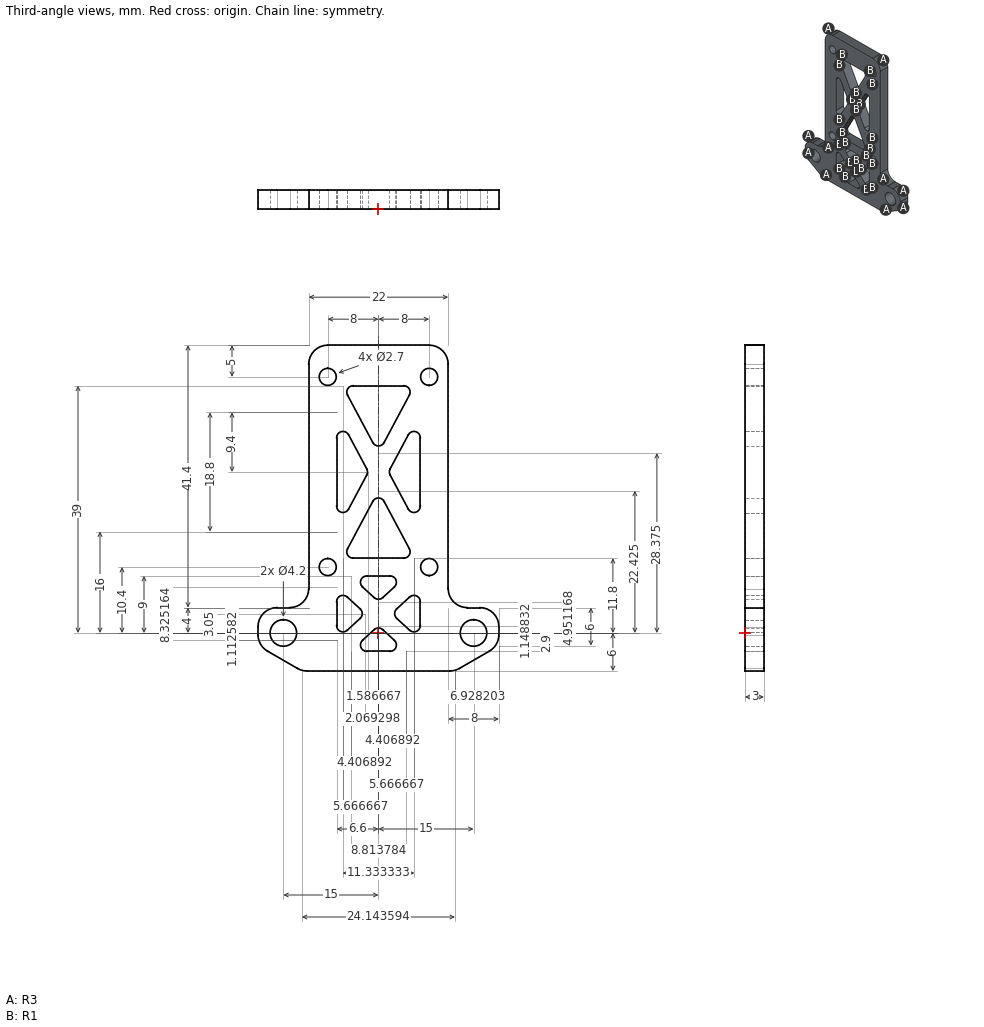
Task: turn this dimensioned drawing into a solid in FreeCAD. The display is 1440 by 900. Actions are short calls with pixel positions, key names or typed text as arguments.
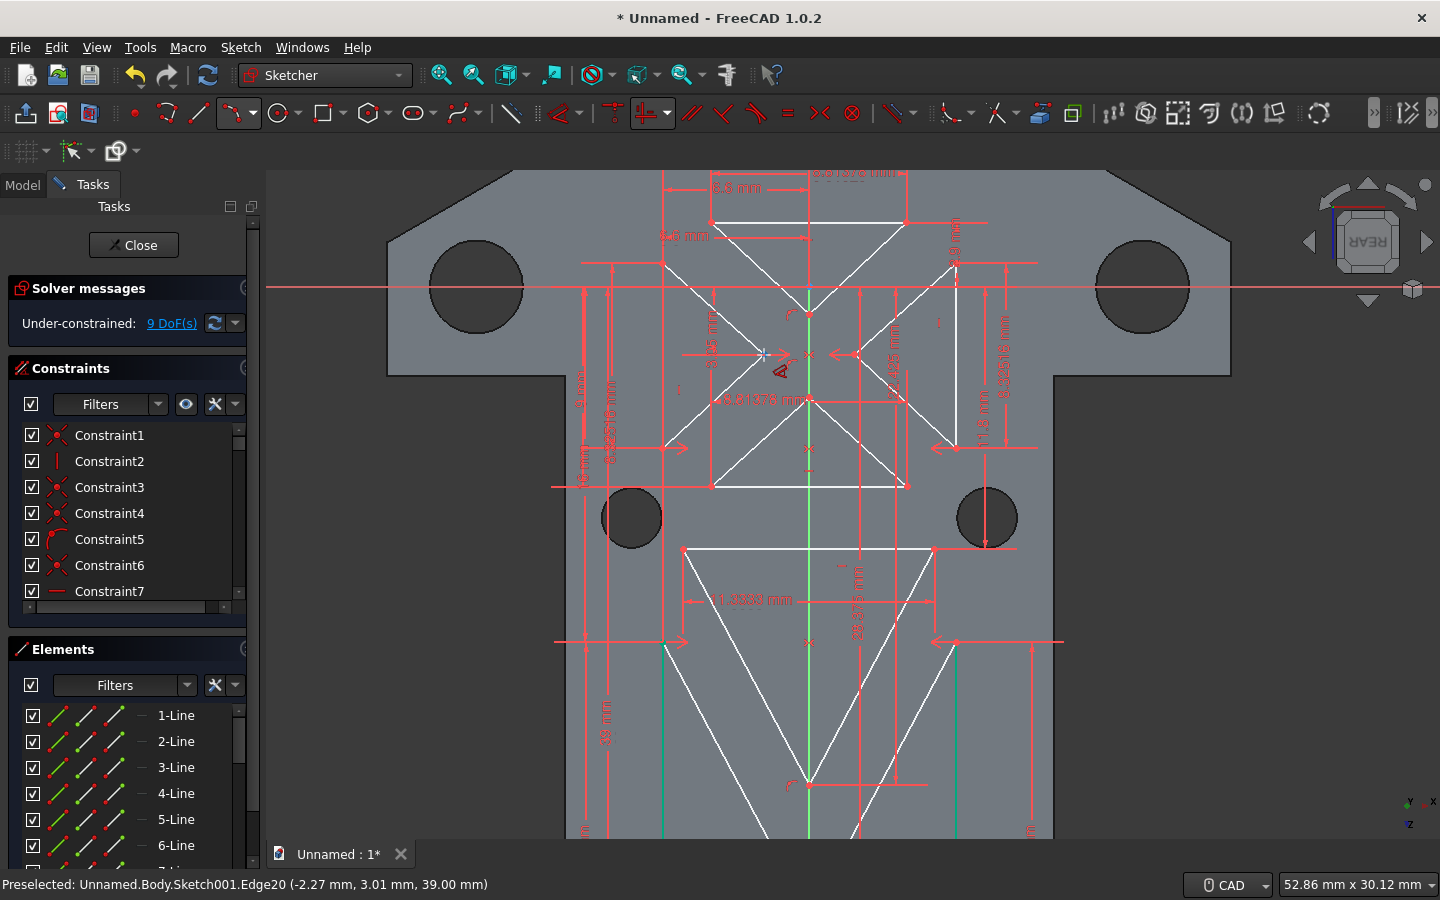
click(764, 355)
click(787, 253)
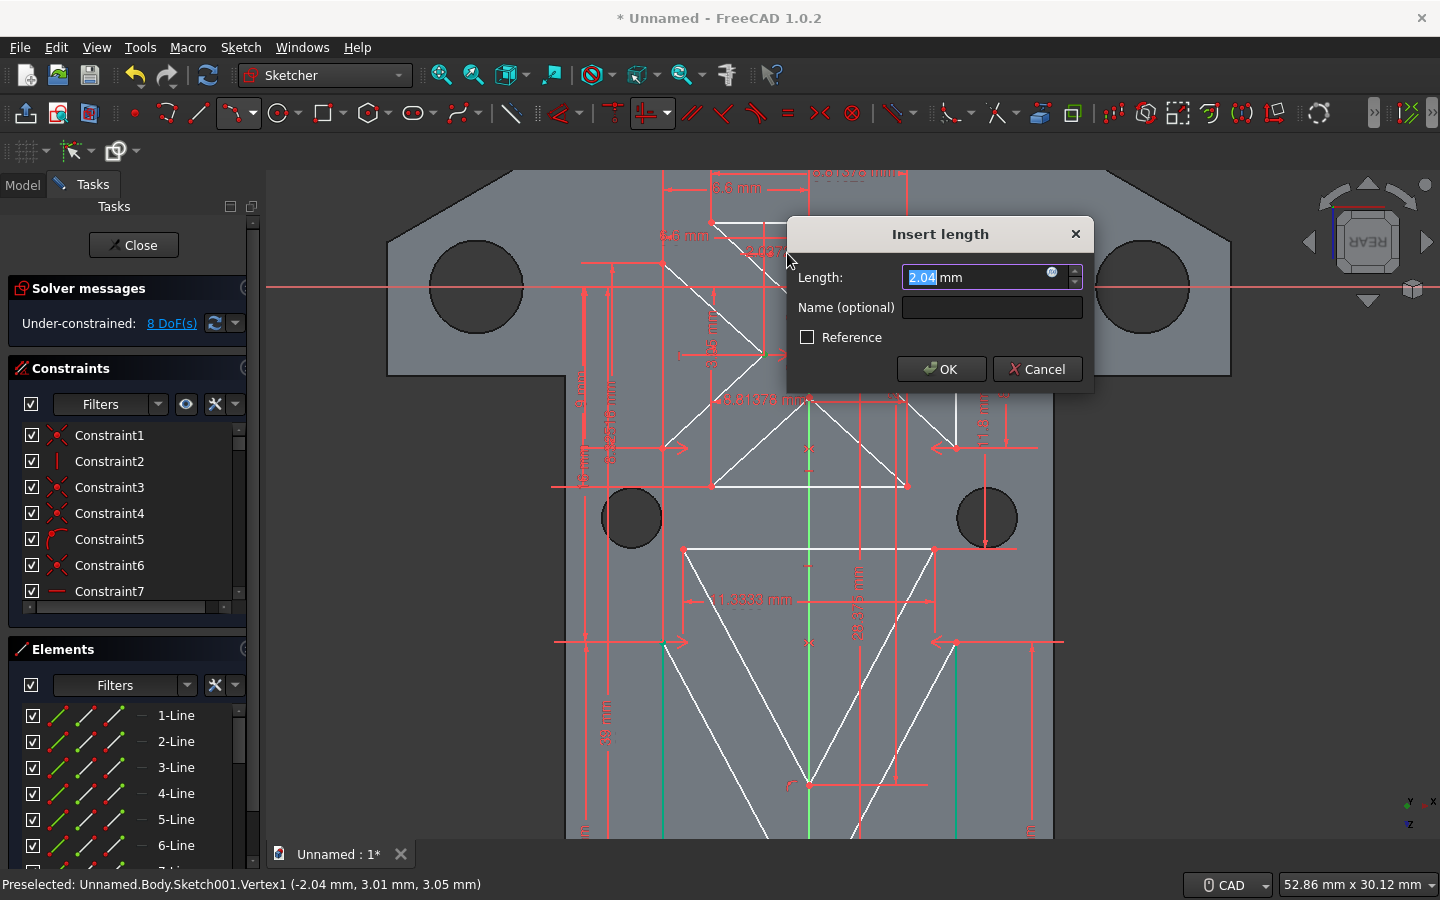
text(2.069298)
key(Return)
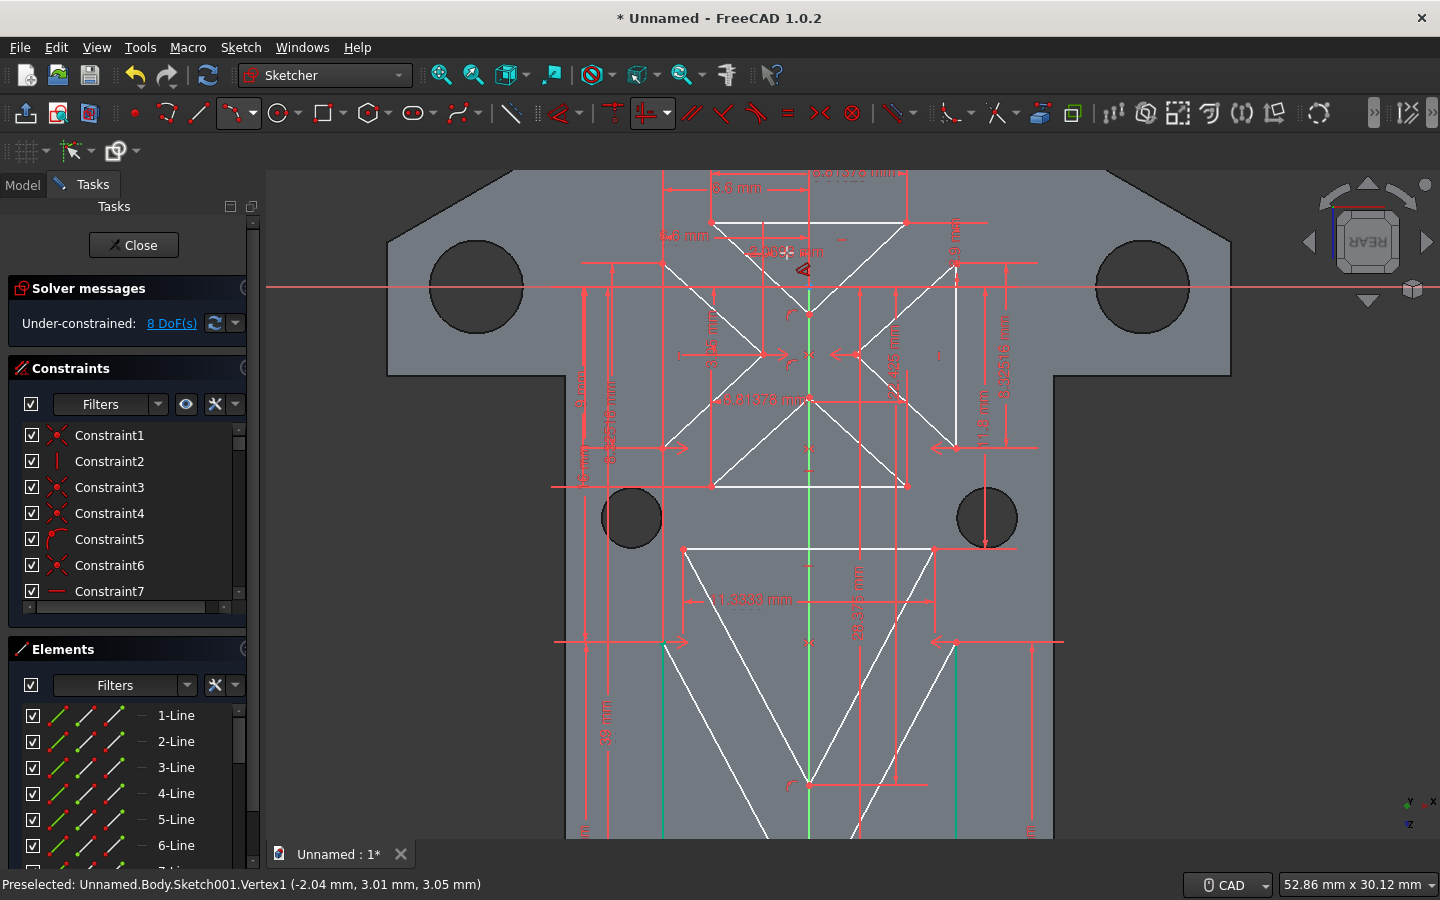
scroll(663, 263, up, 3)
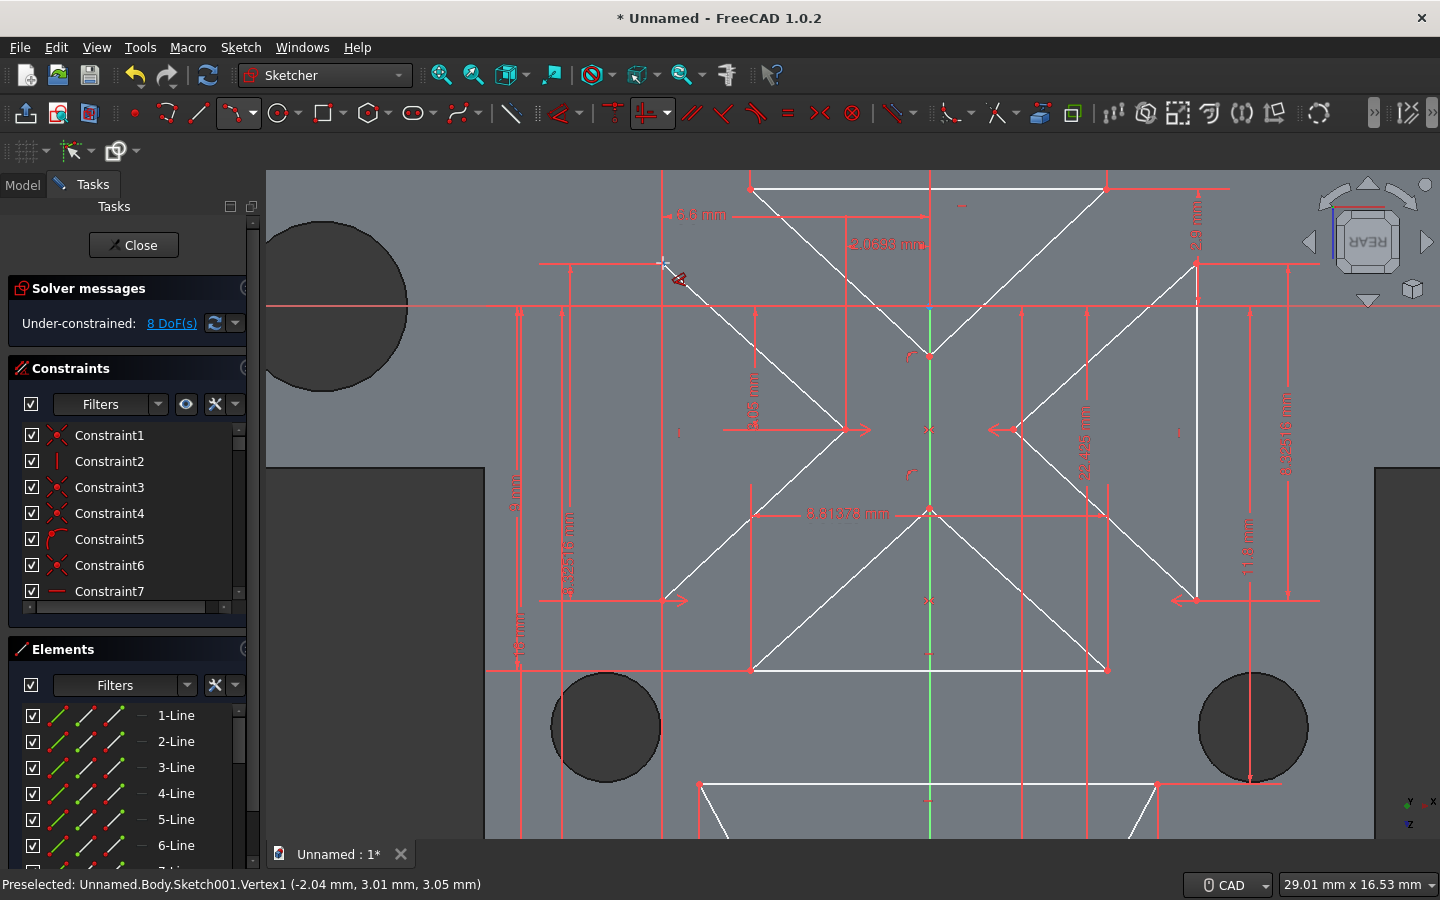
click(662, 264)
click(628, 285)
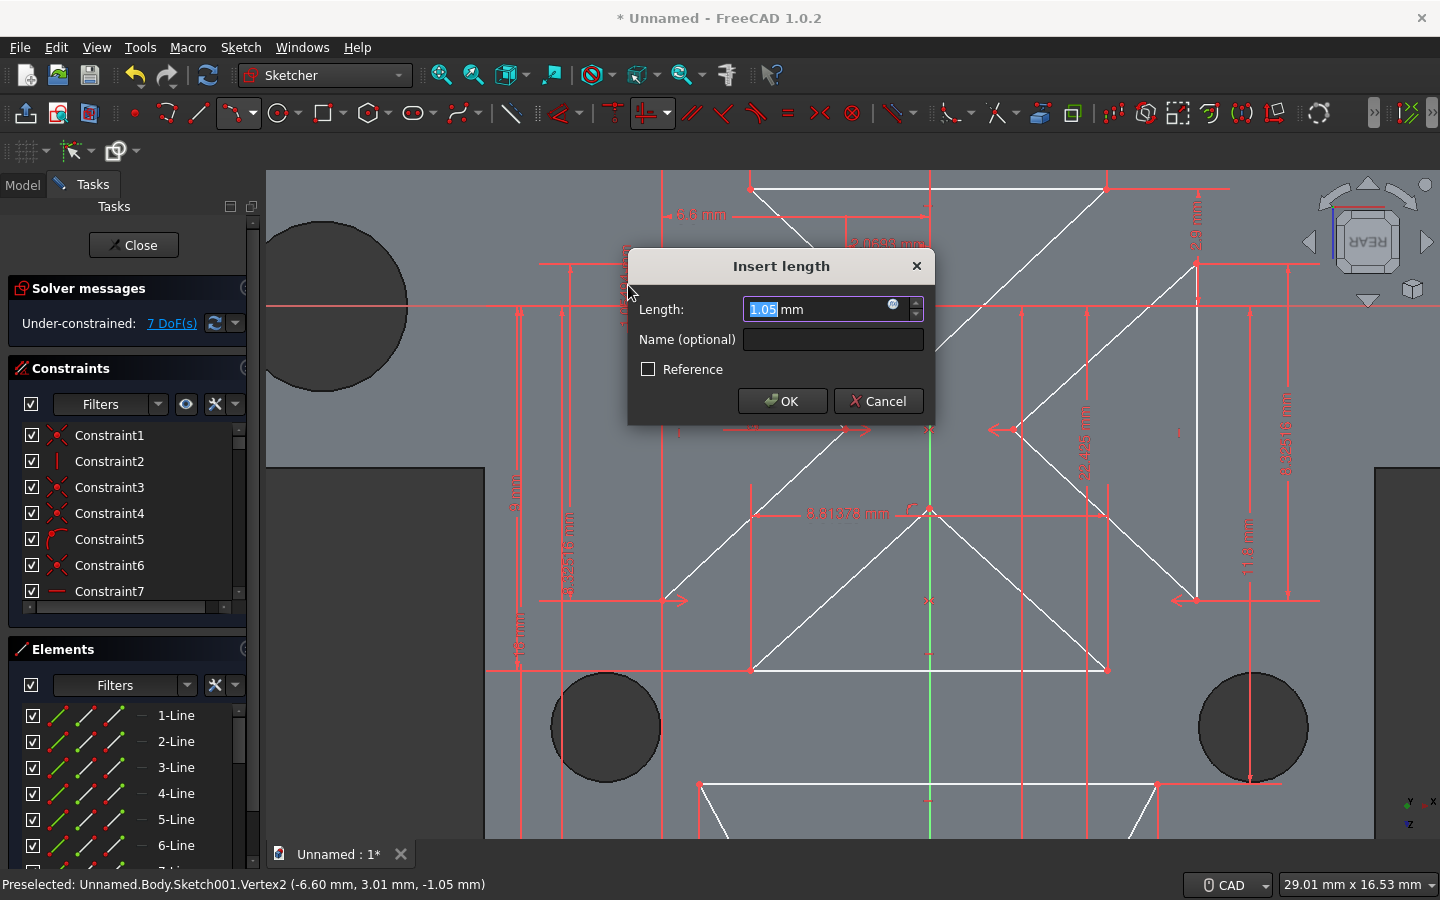
text(1.112582)
key(Return)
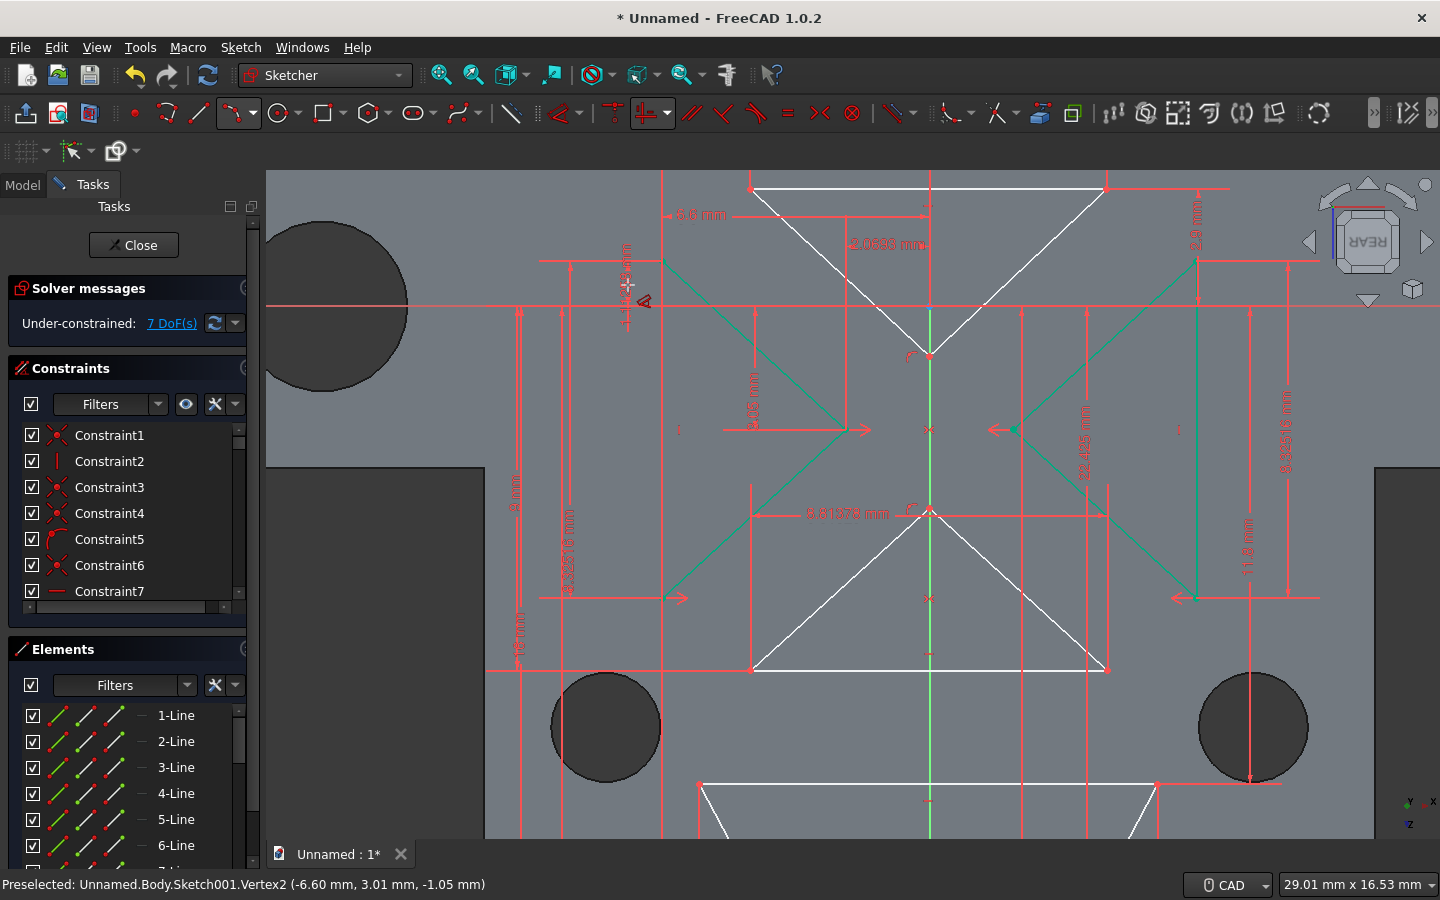
click(930, 356)
click(964, 343)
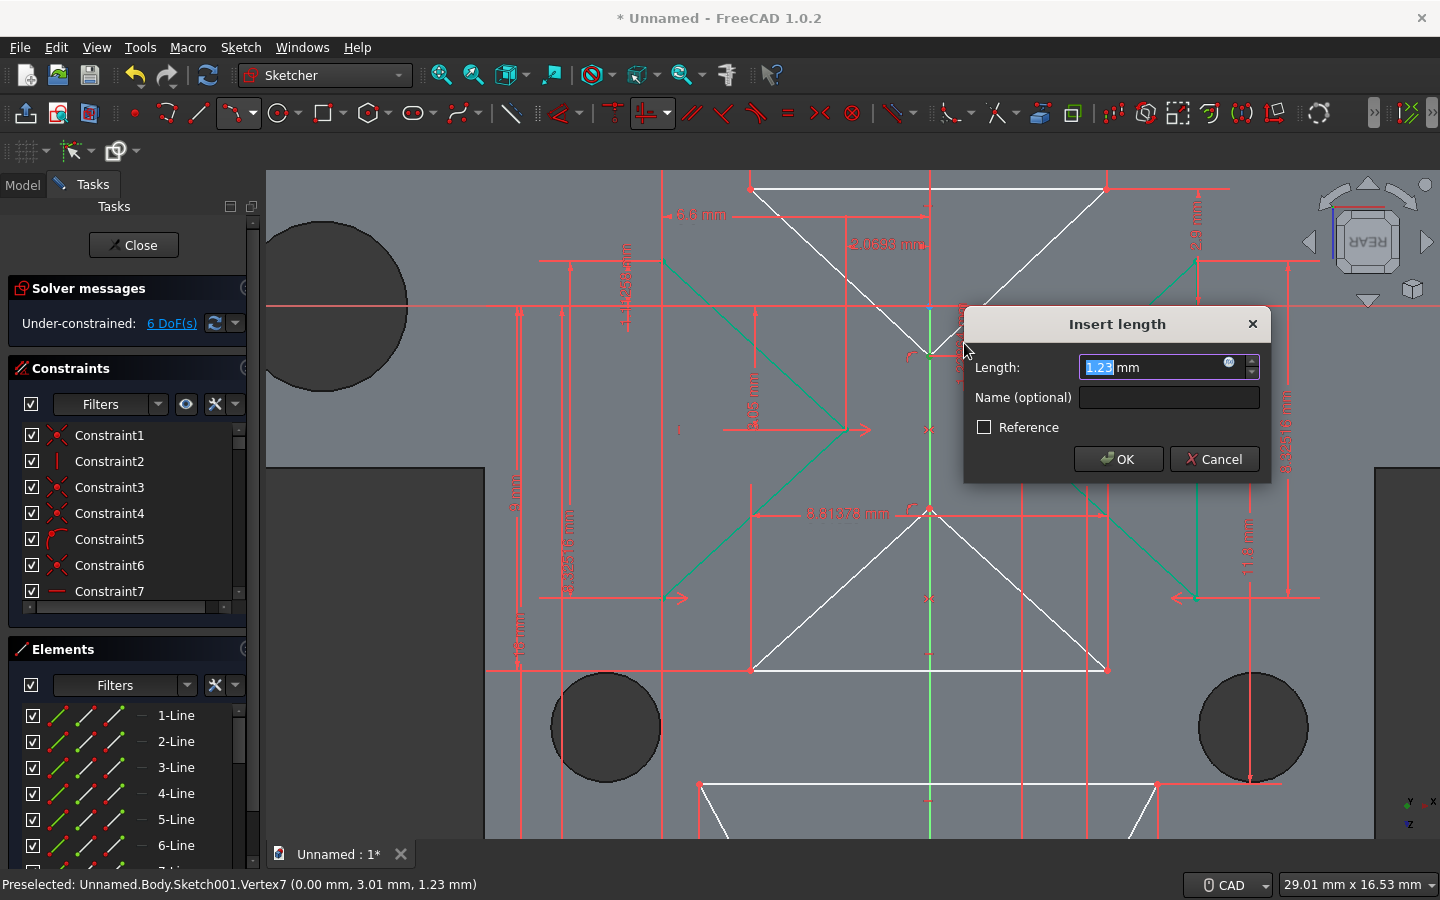
text(1.148832)
key(Return)